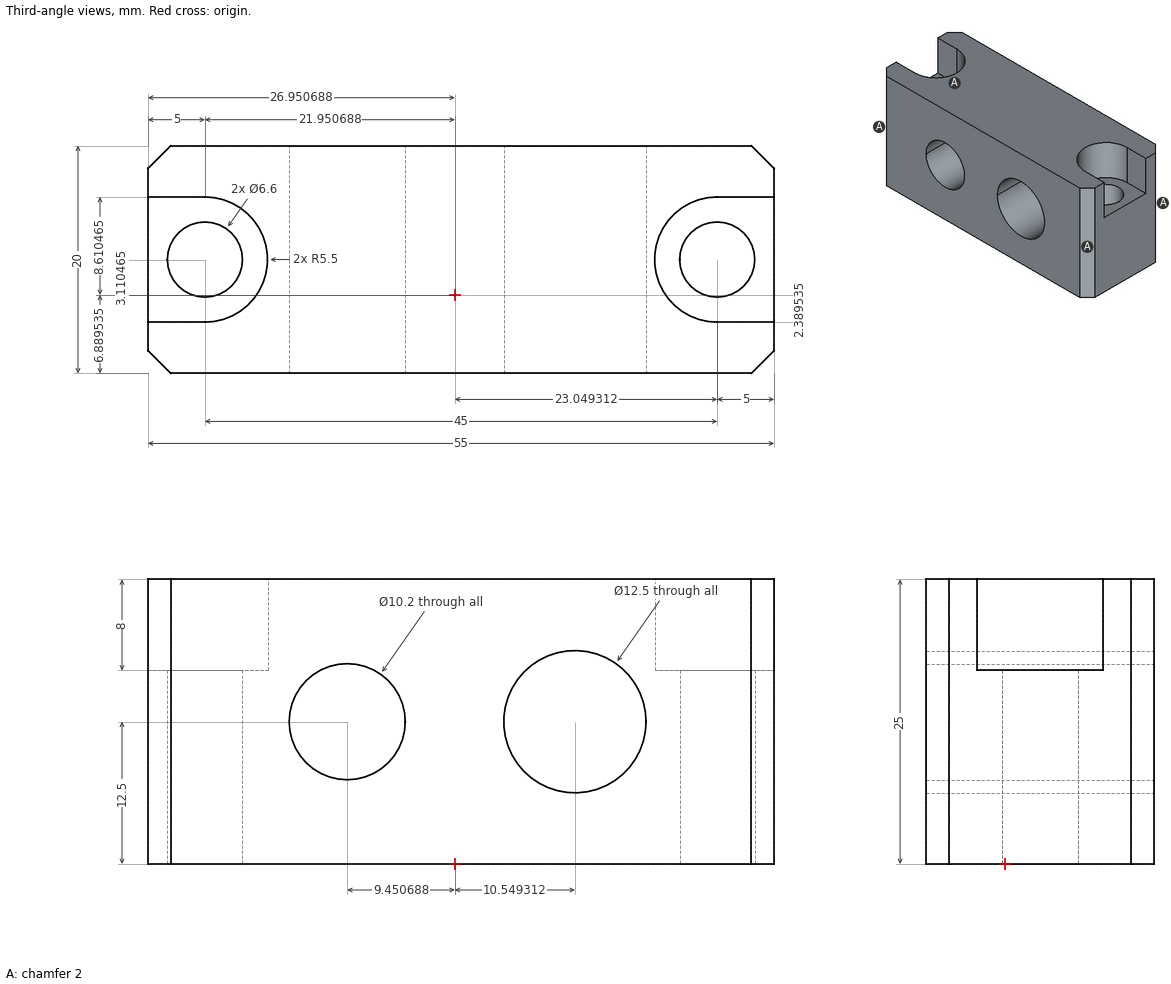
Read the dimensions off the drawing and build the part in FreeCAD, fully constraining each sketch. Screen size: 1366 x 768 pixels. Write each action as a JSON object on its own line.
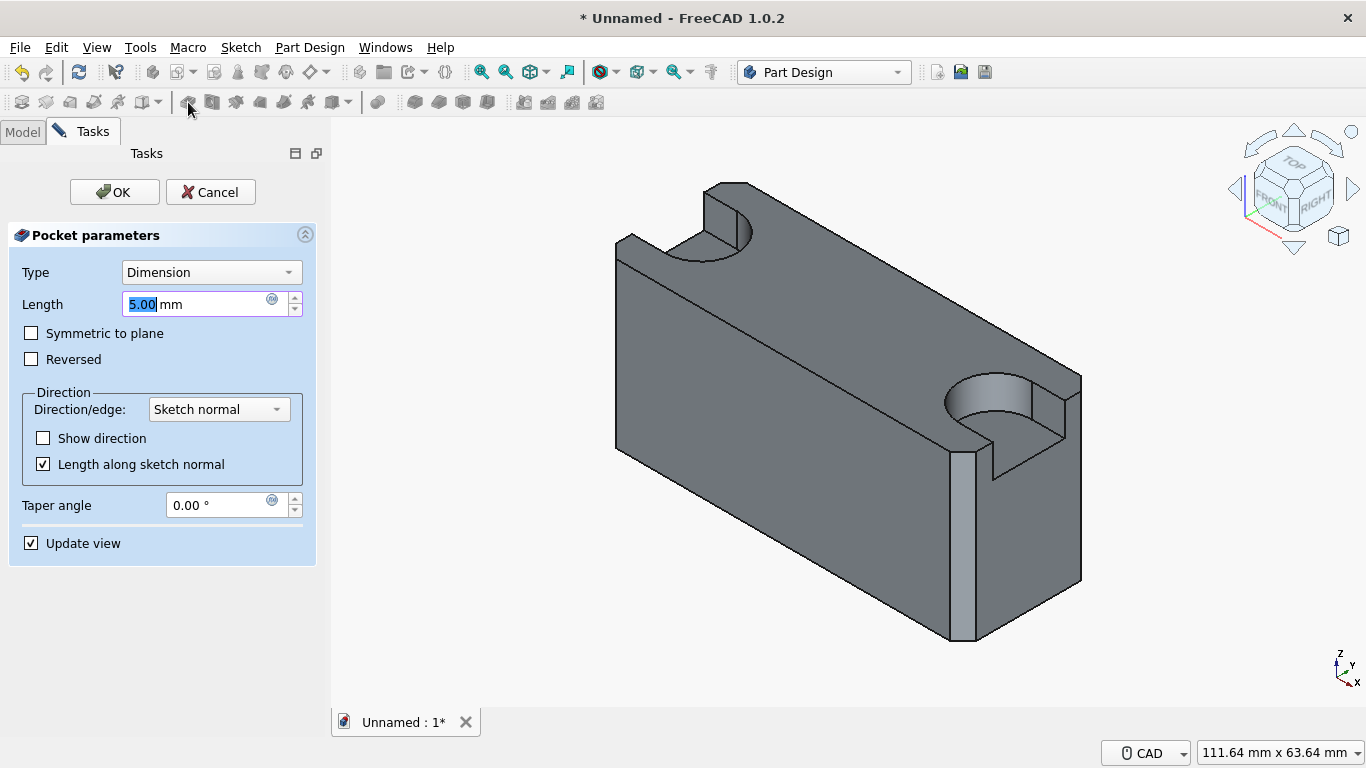
{"action": "type", "text": "8"}
{"action": "key", "text": "Tab"}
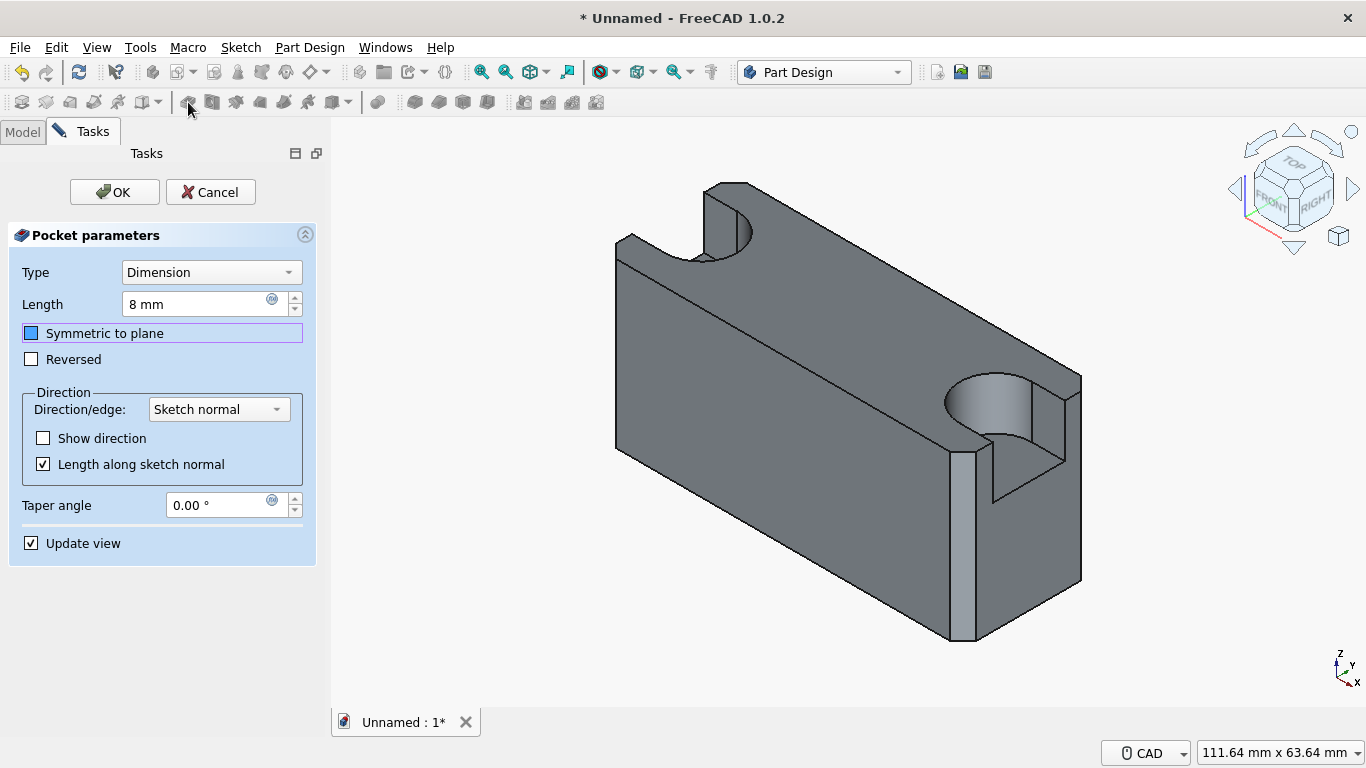
{"action": "left_click", "coordinate": [115, 192]}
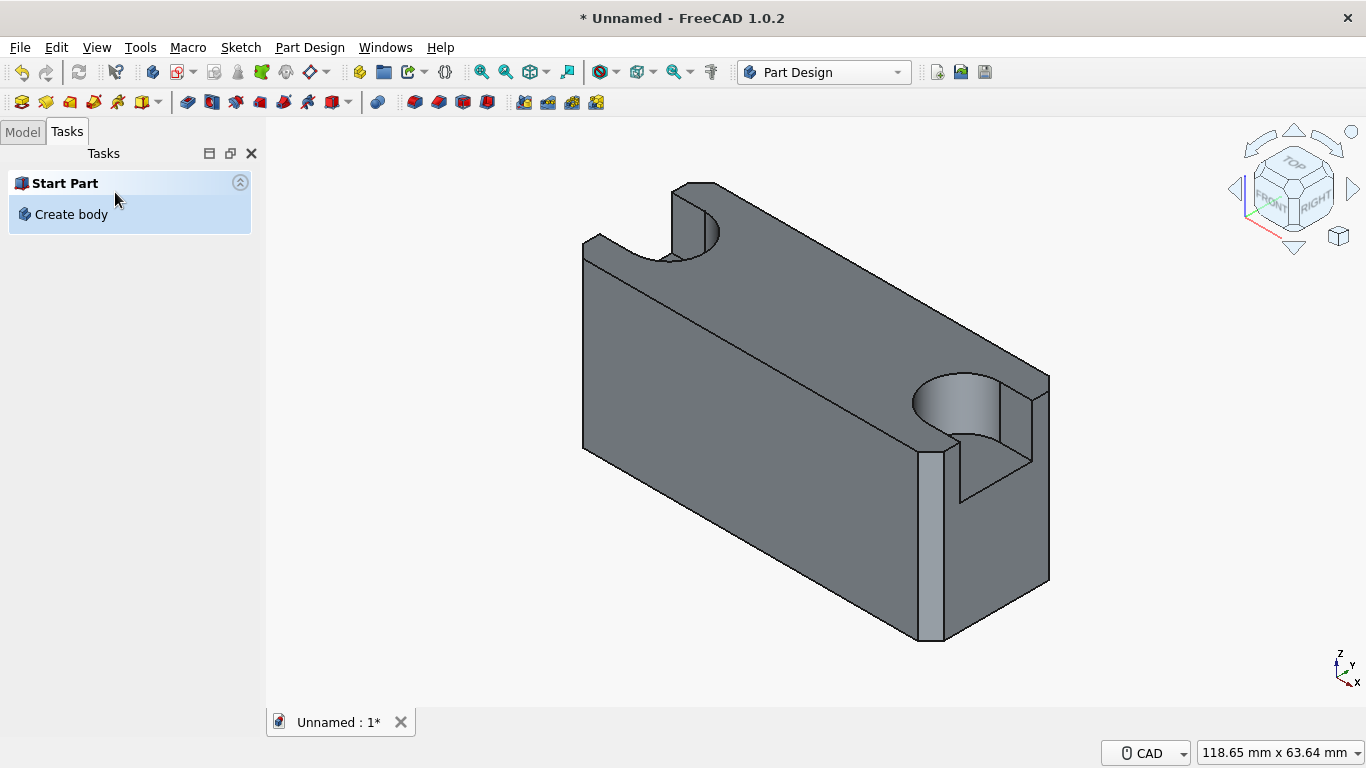
{"action": "left_click", "coordinate": [972, 455]}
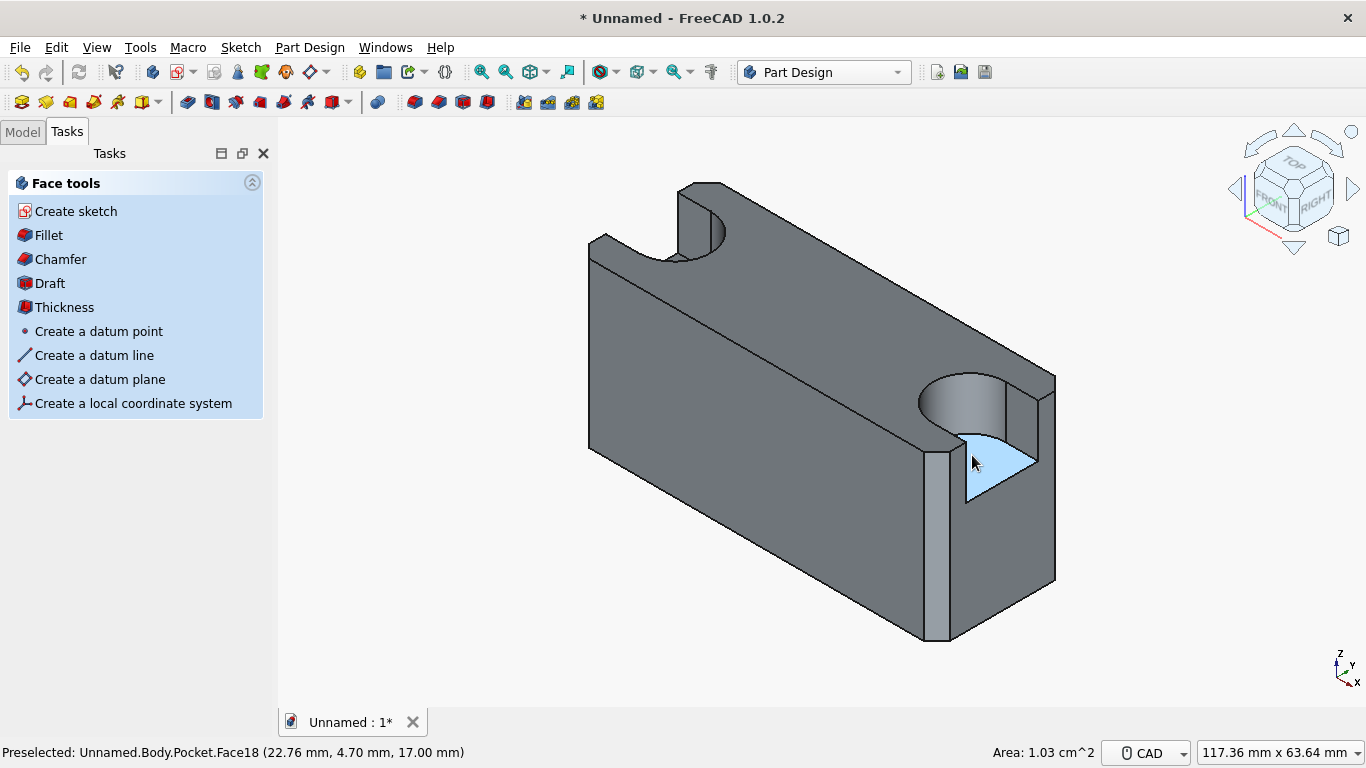
{"action": "left_click", "coordinate": [178, 72]}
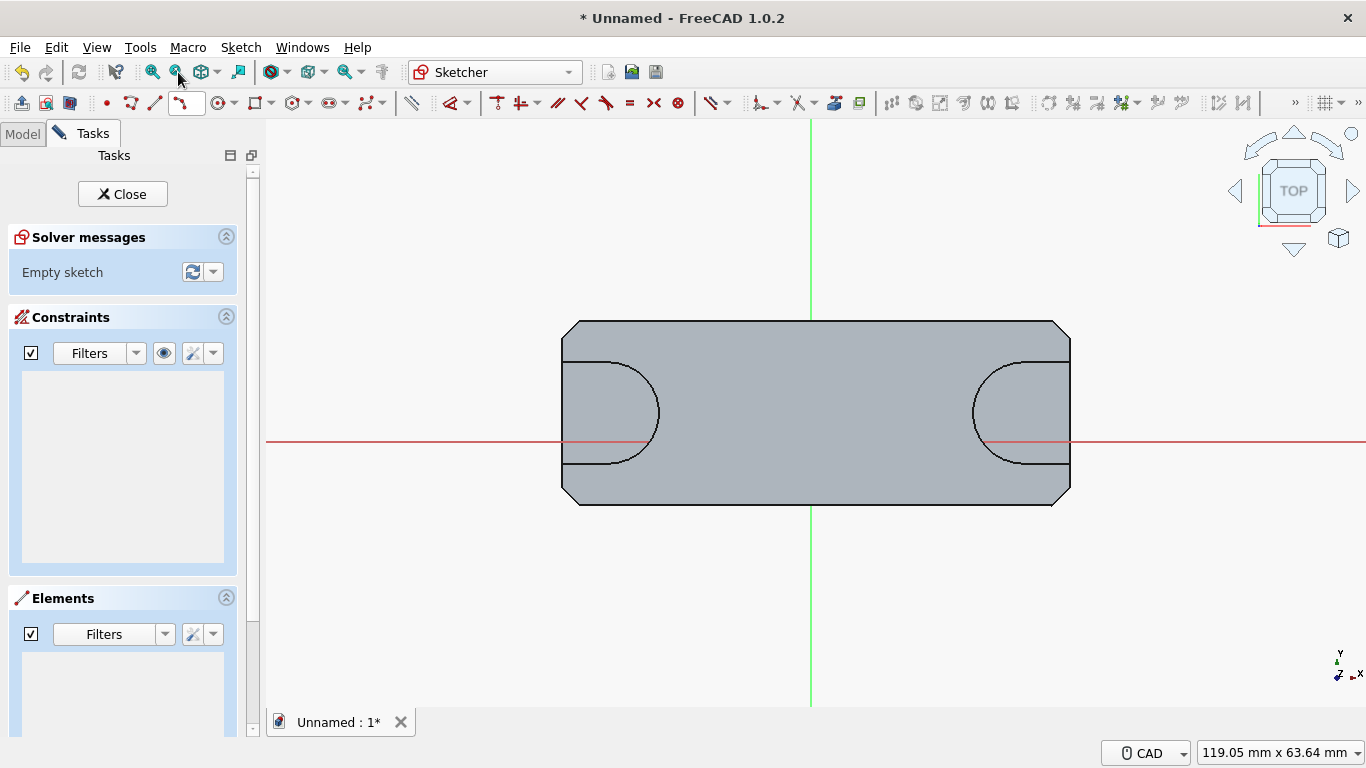
{"action": "left_click", "coordinate": [70, 104]}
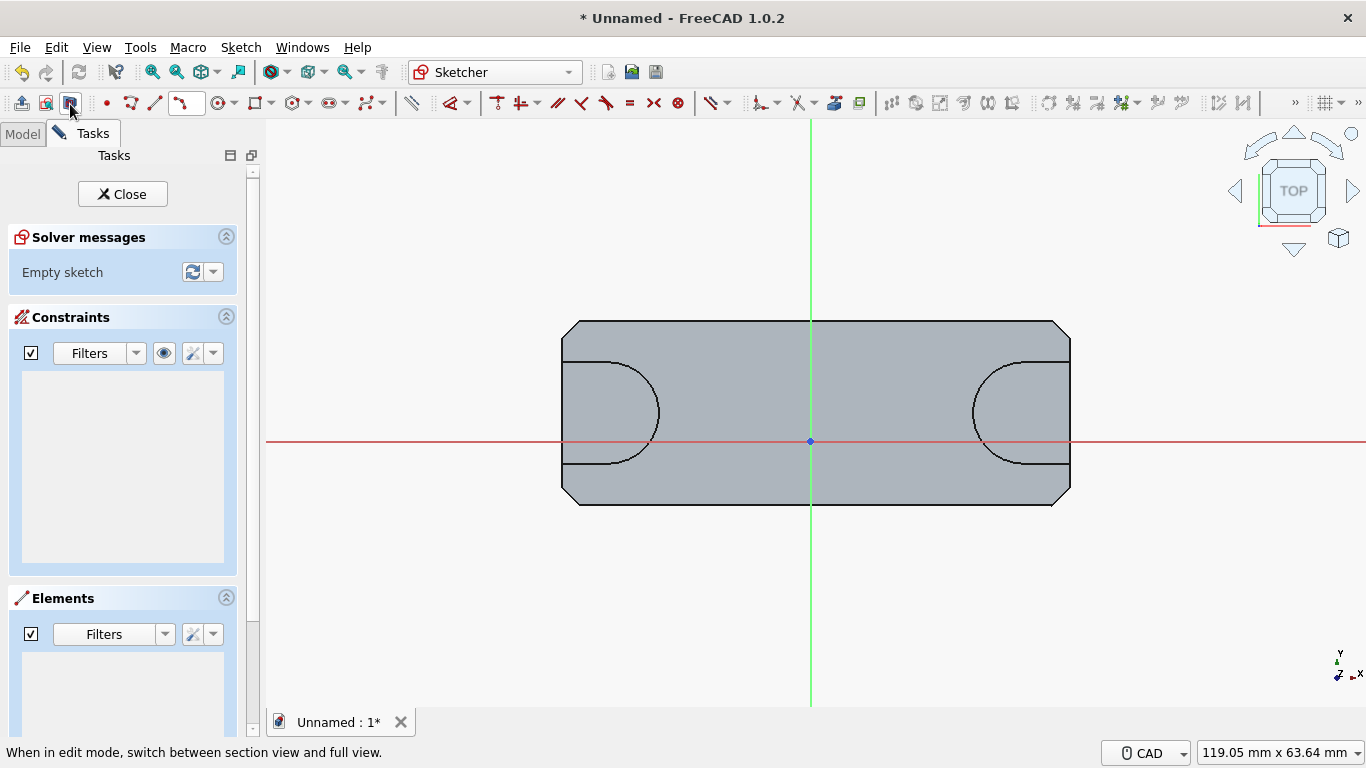
{"action": "key", "text": "g c"}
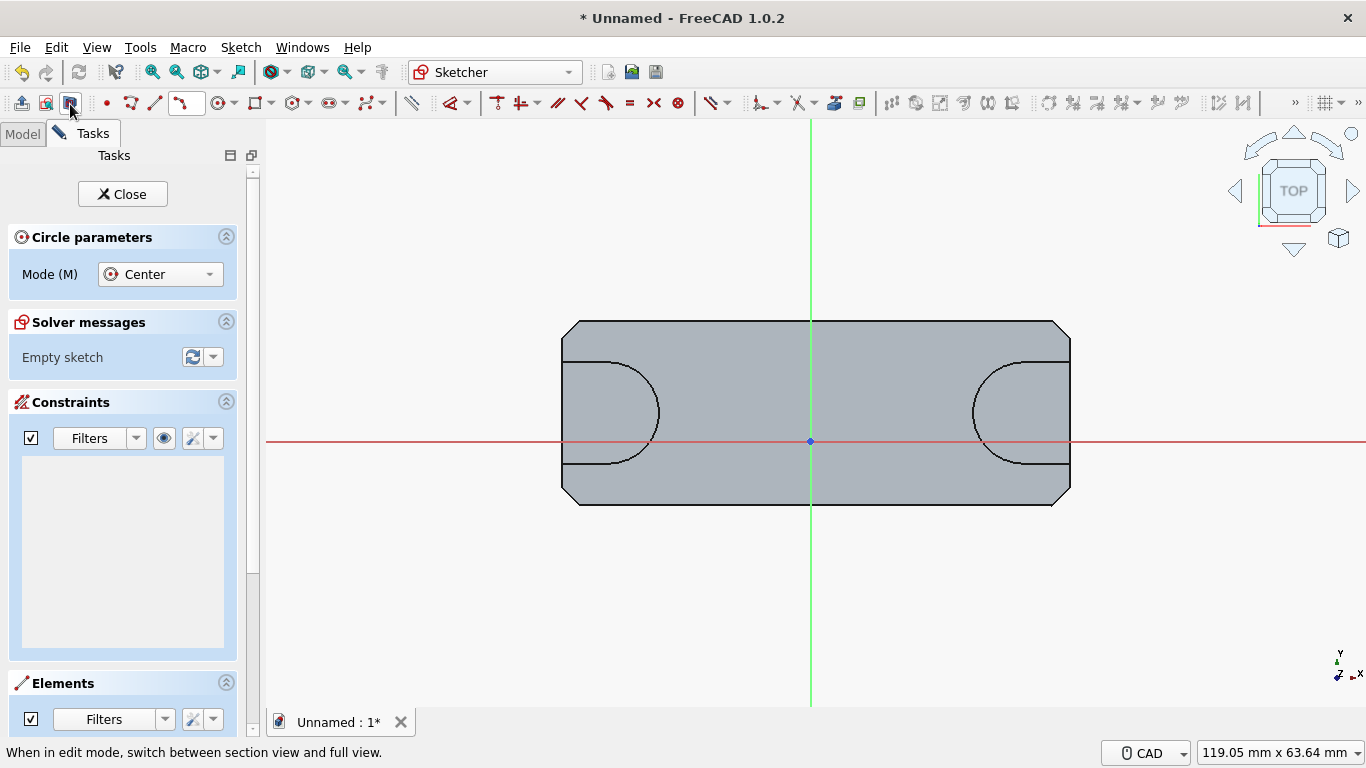
{"action": "left_click", "coordinate": [608, 413]}
{"action": "left_click", "coordinate": [630, 391]}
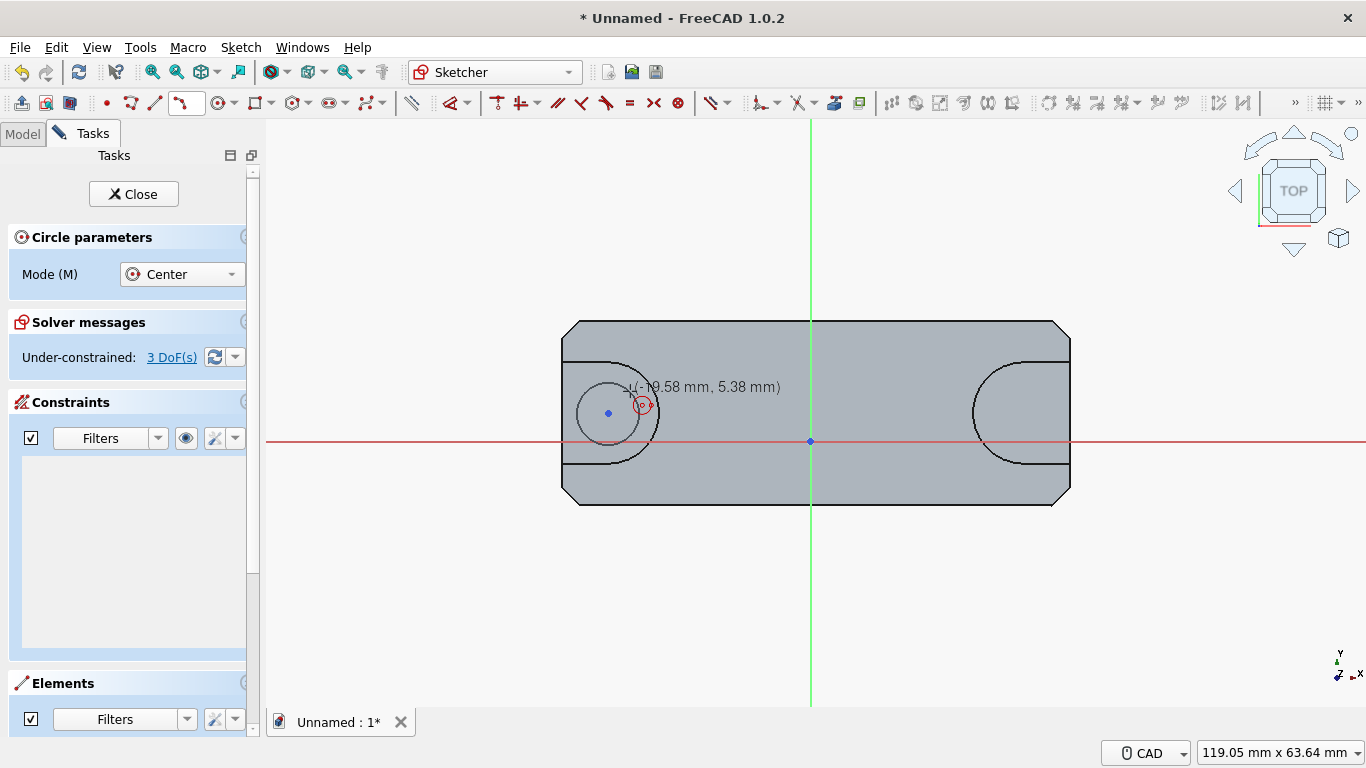
{"action": "left_click", "coordinate": [1024, 413]}
{"action": "left_click", "coordinate": [1045, 391]}
{"action": "key", "text": "Escape"}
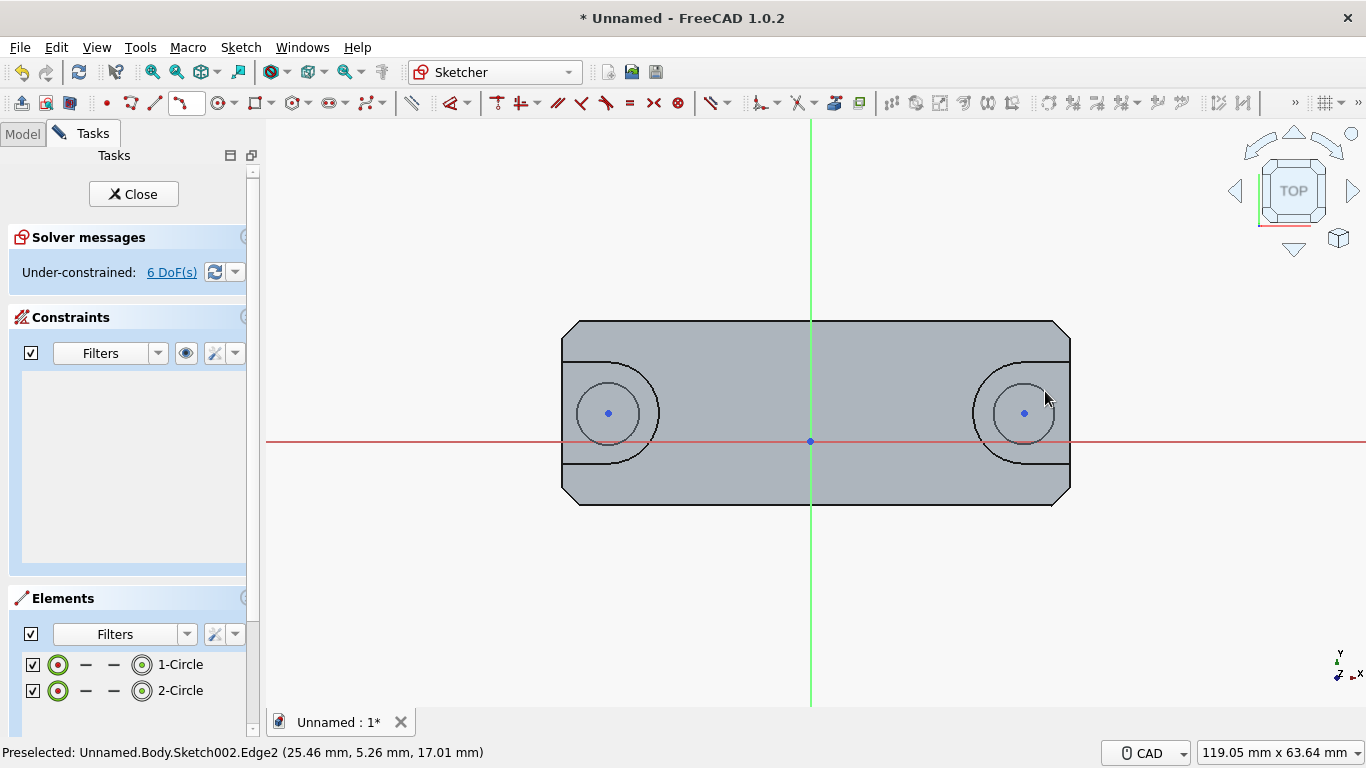
{"action": "left_click", "coordinate": [630, 392]}